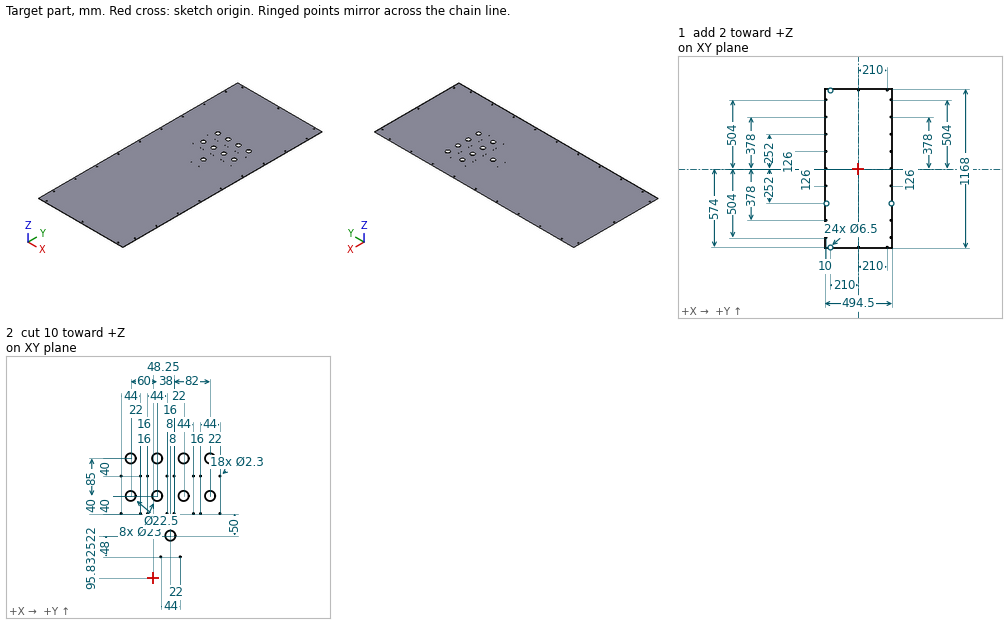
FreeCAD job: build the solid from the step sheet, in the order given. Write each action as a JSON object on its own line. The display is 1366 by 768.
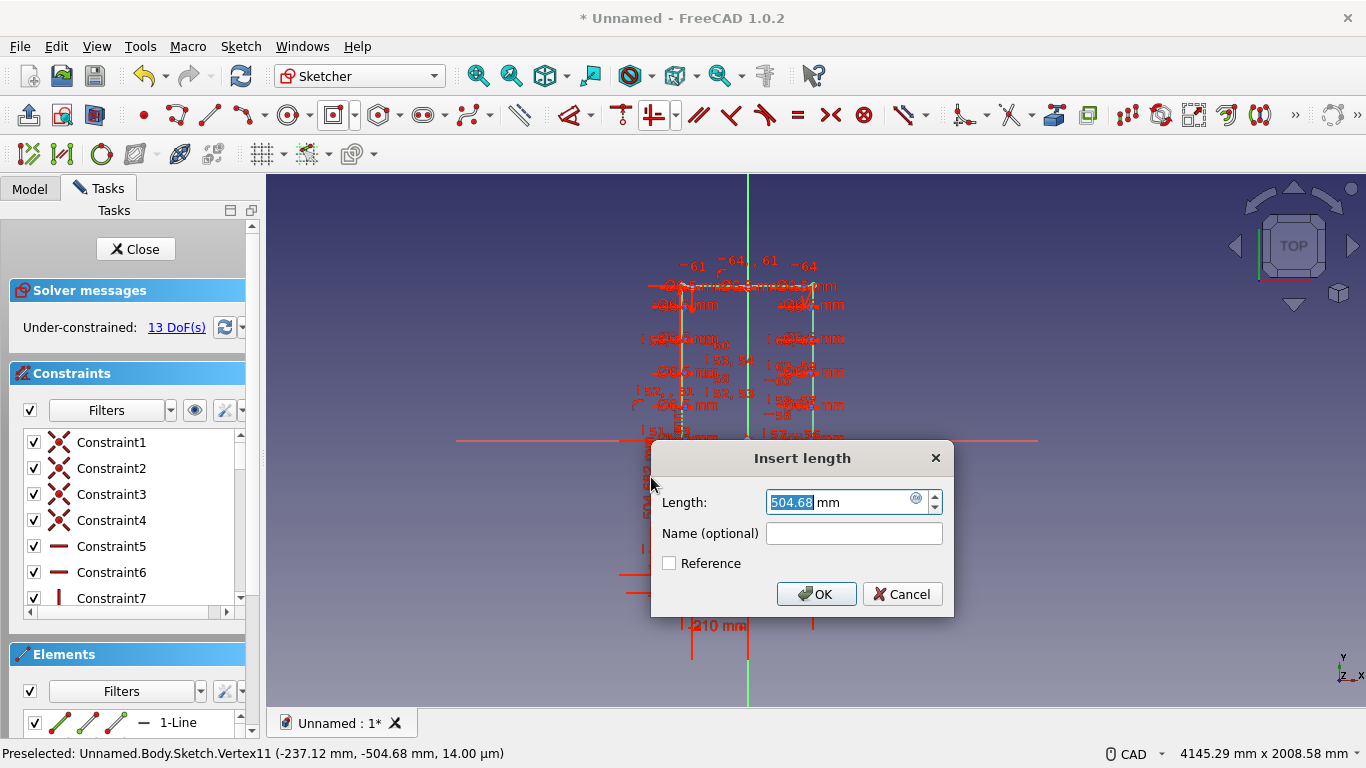
{"action": "type", "text": "504"}
{"action": "key", "text": "Return"}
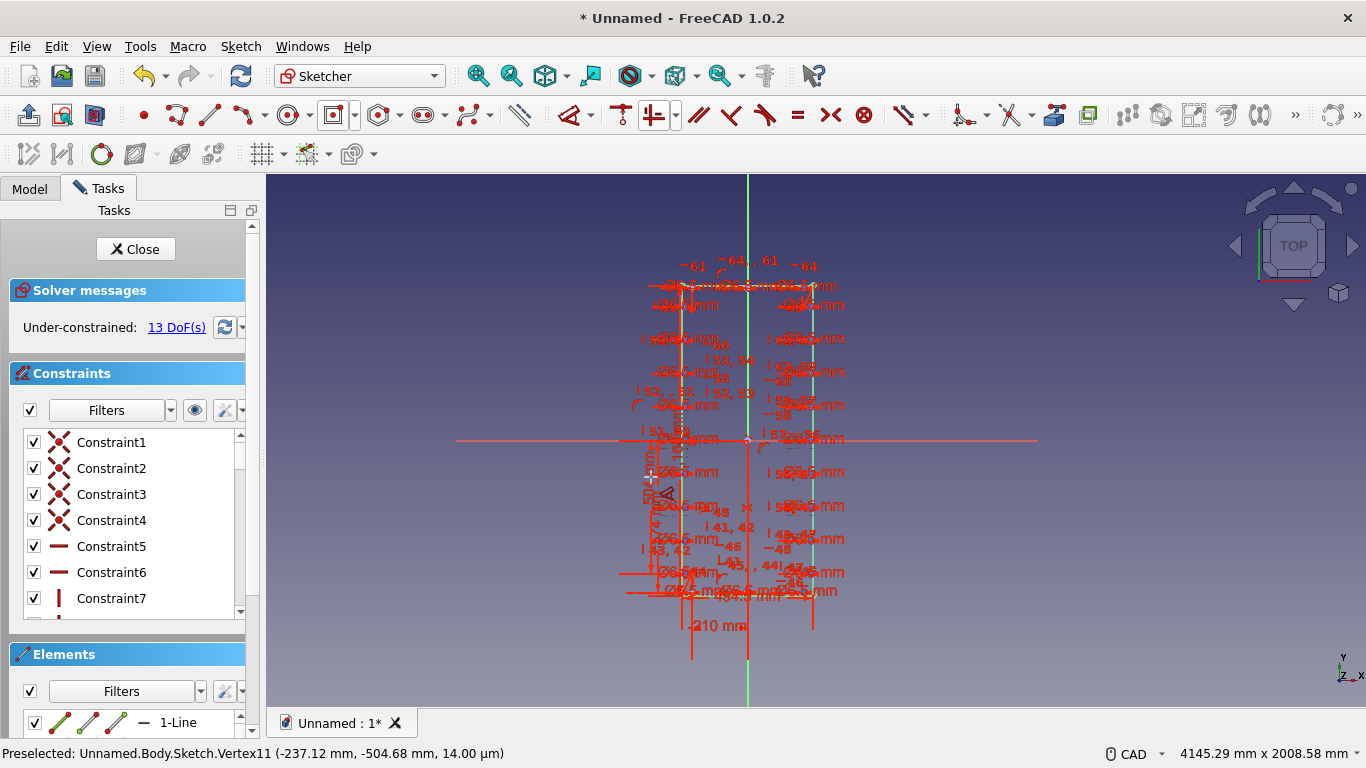
{"action": "left_click", "coordinate": [685, 541]}
{"action": "left_click", "coordinate": [651, 456]}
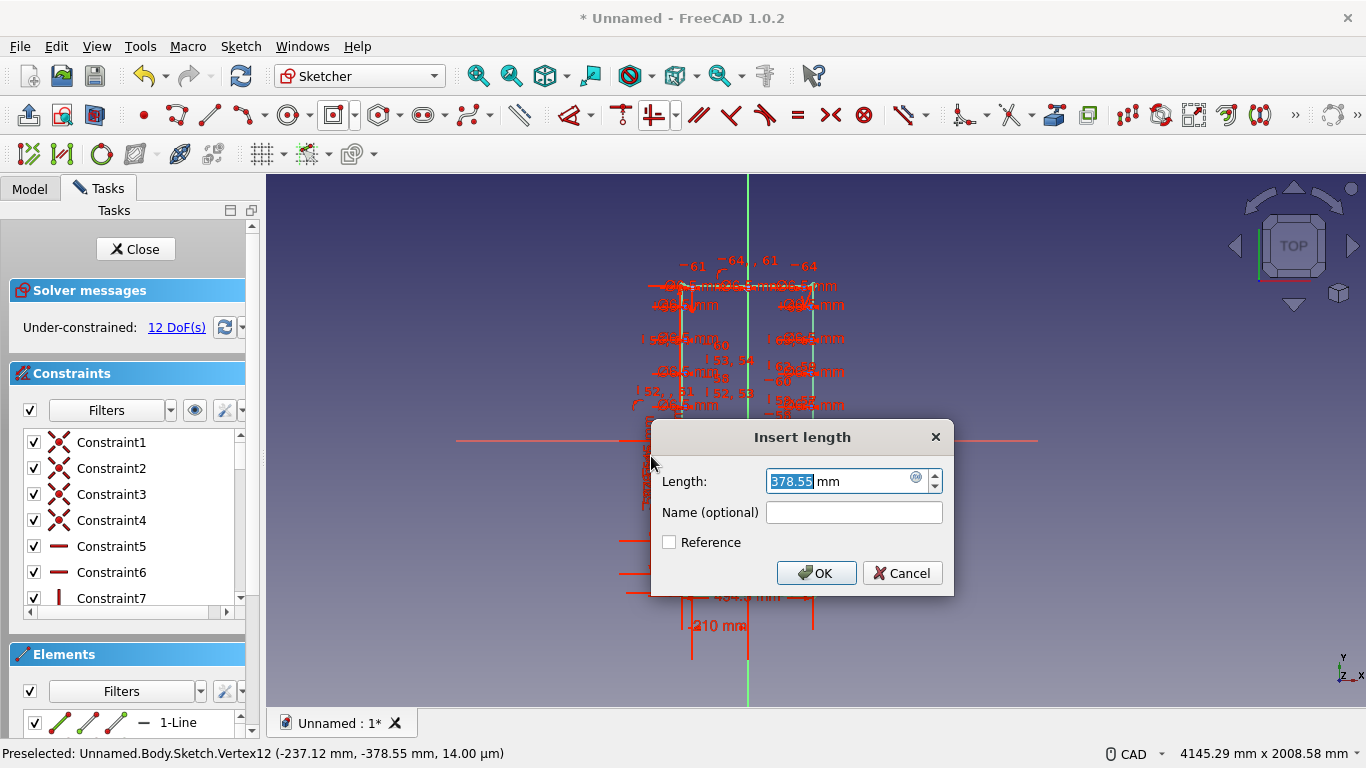
{"action": "type", "text": "378"}
{"action": "key", "text": "Return"}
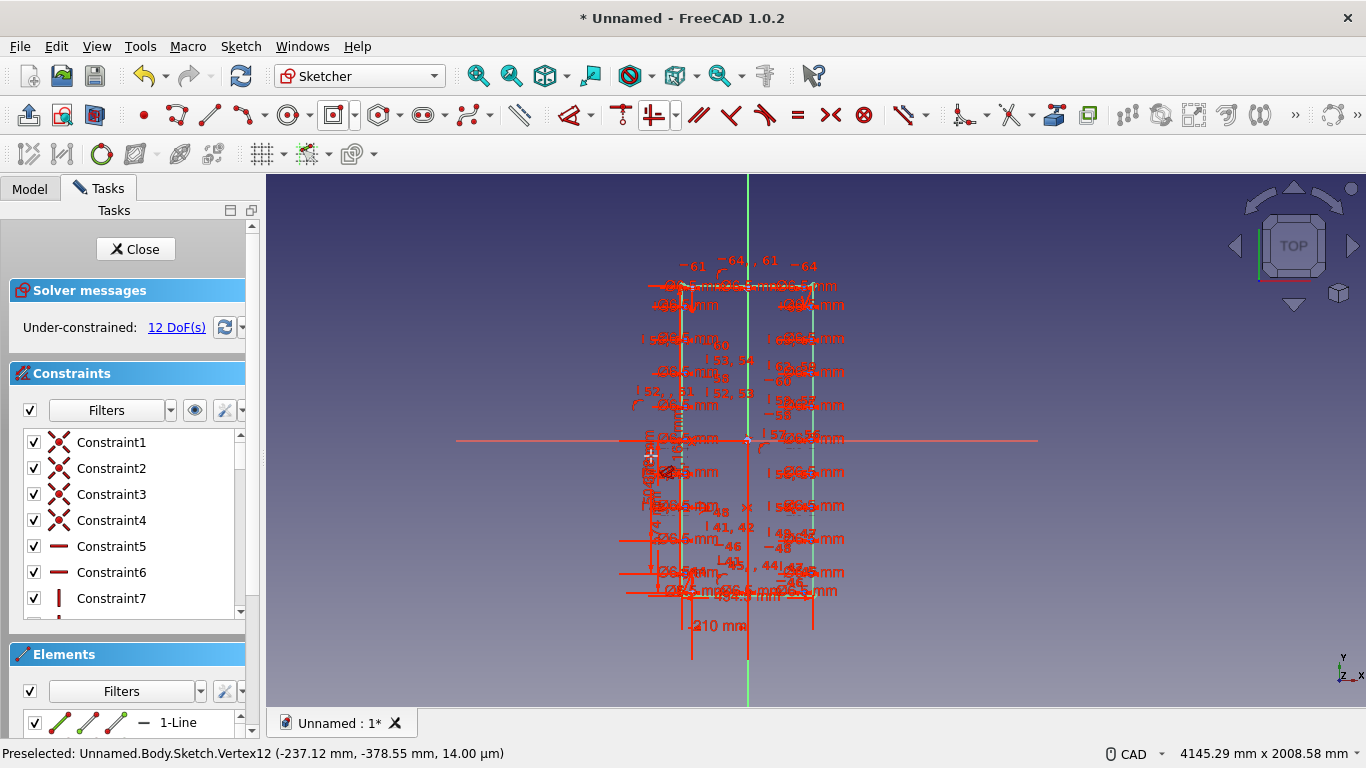
{"action": "left_click", "coordinate": [685, 508]}
{"action": "left_click", "coordinate": [782, 474]}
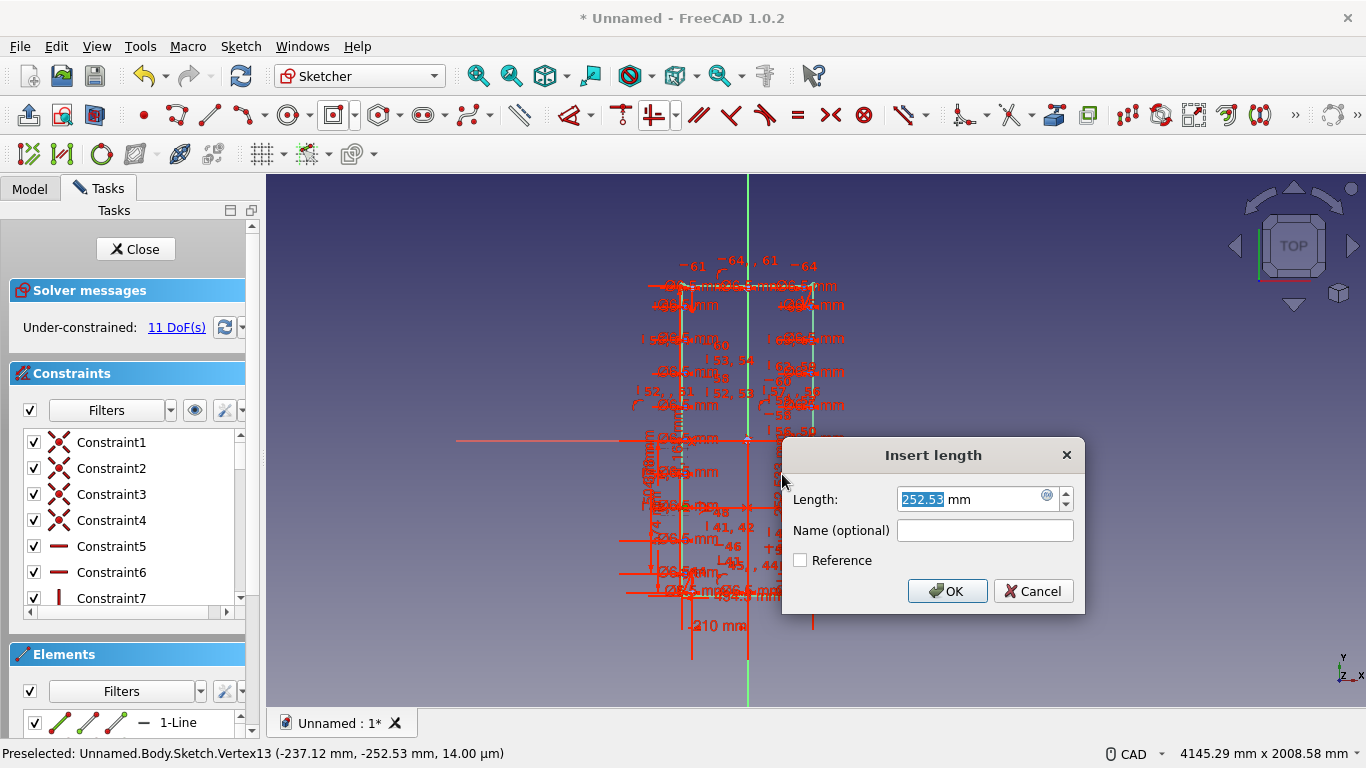
{"action": "type", "text": "252"}
{"action": "key", "text": "Return"}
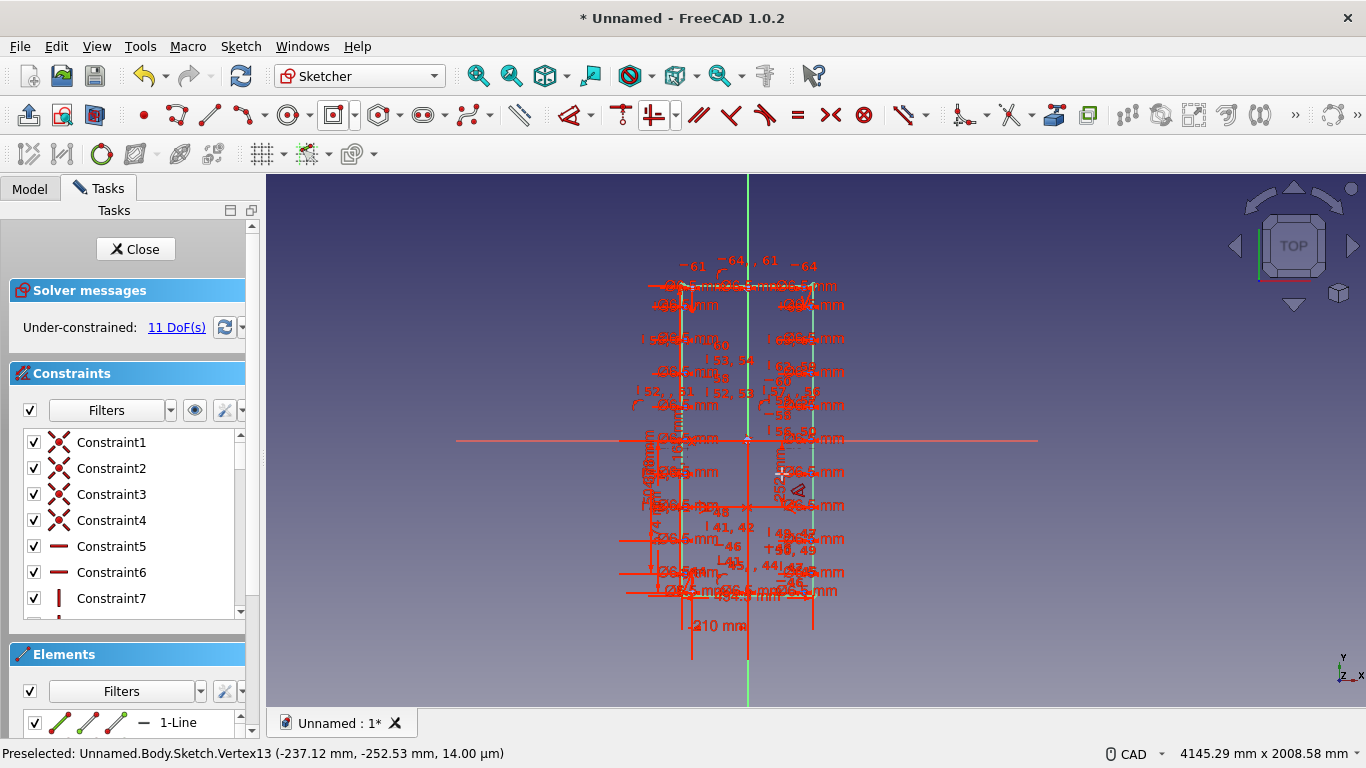
{"action": "left_click", "coordinate": [685, 474]}
{"action": "left_click", "coordinate": [579, 457]}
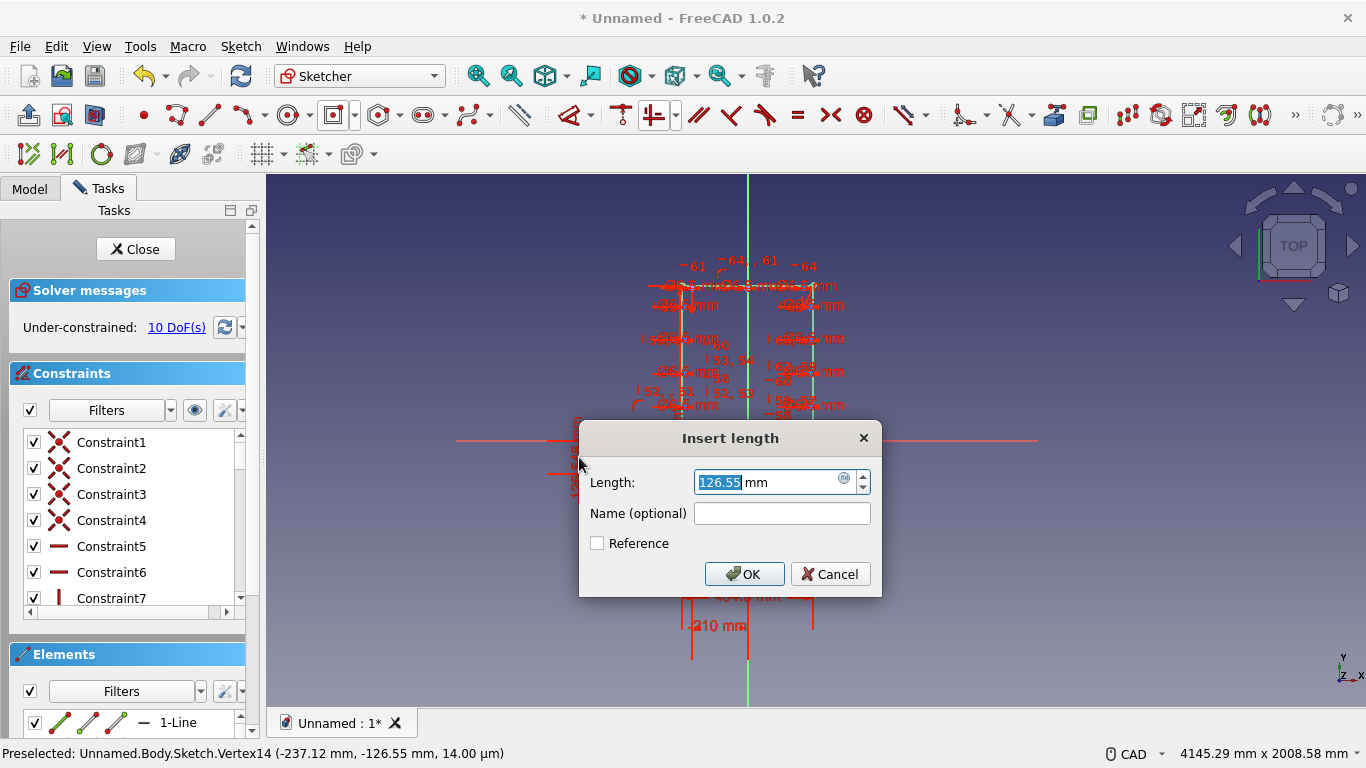
{"action": "type", "text": "126"}
{"action": "key", "text": "Return"}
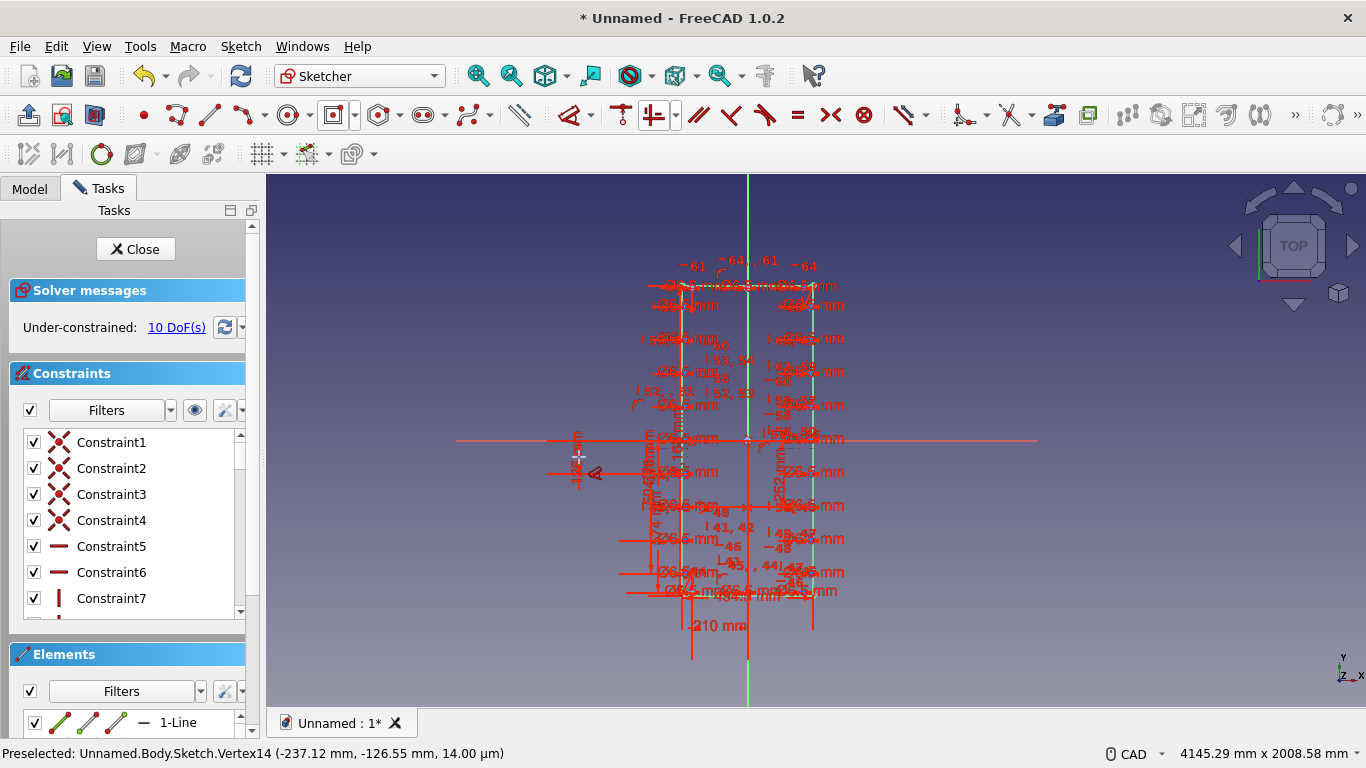
{"action": "left_click", "coordinate": [804, 593]}
{"action": "left_click", "coordinate": [795, 627]}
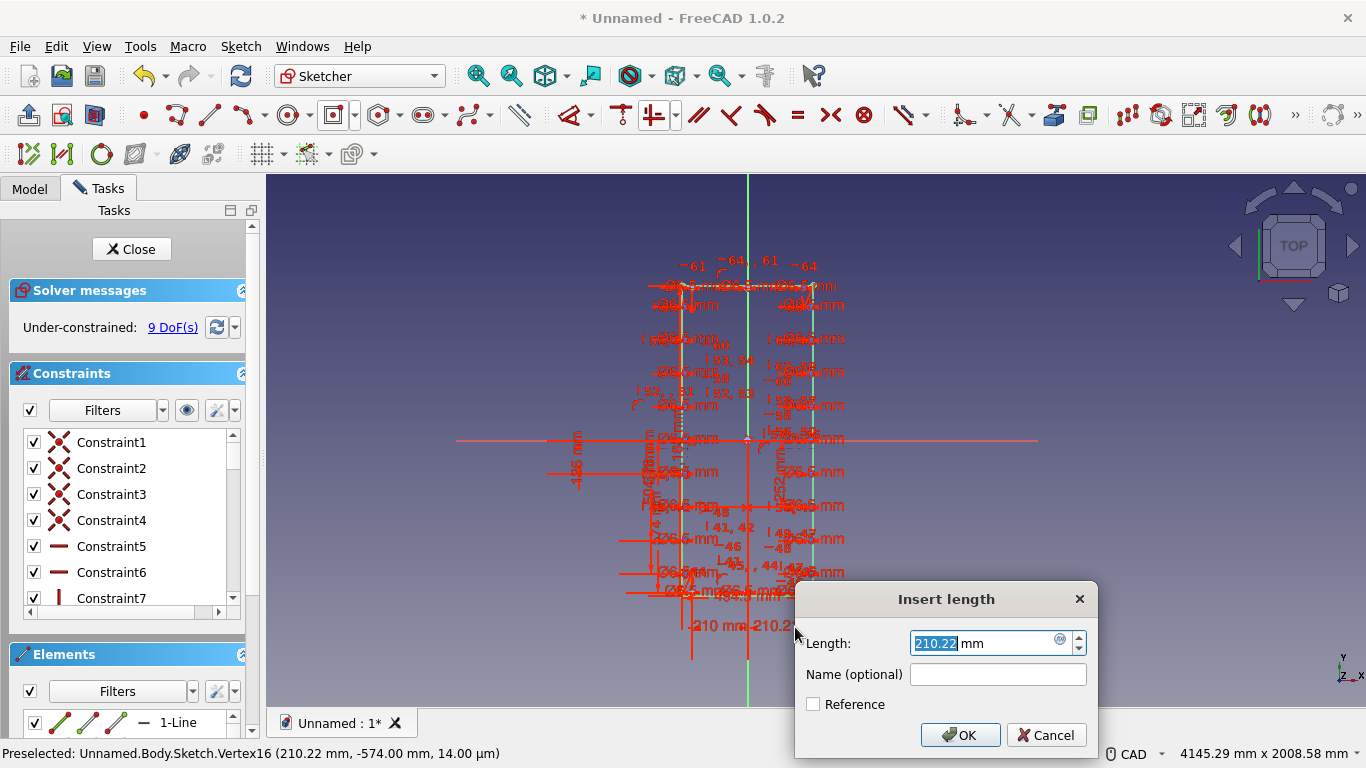
{"action": "type", "text": "210"}
{"action": "key", "text": "Return"}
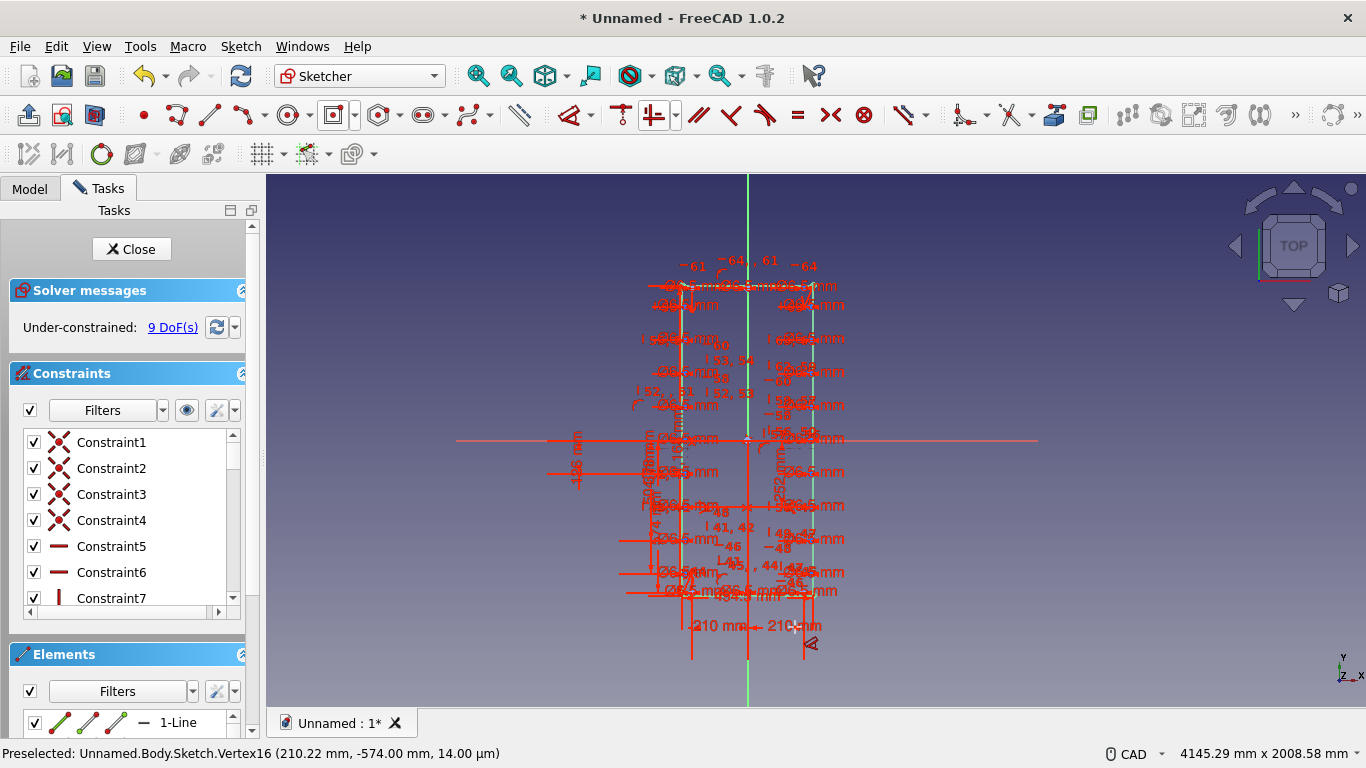
{"action": "left_click", "coordinate": [811, 474]}
{"action": "left_click", "coordinate": [869, 457]}